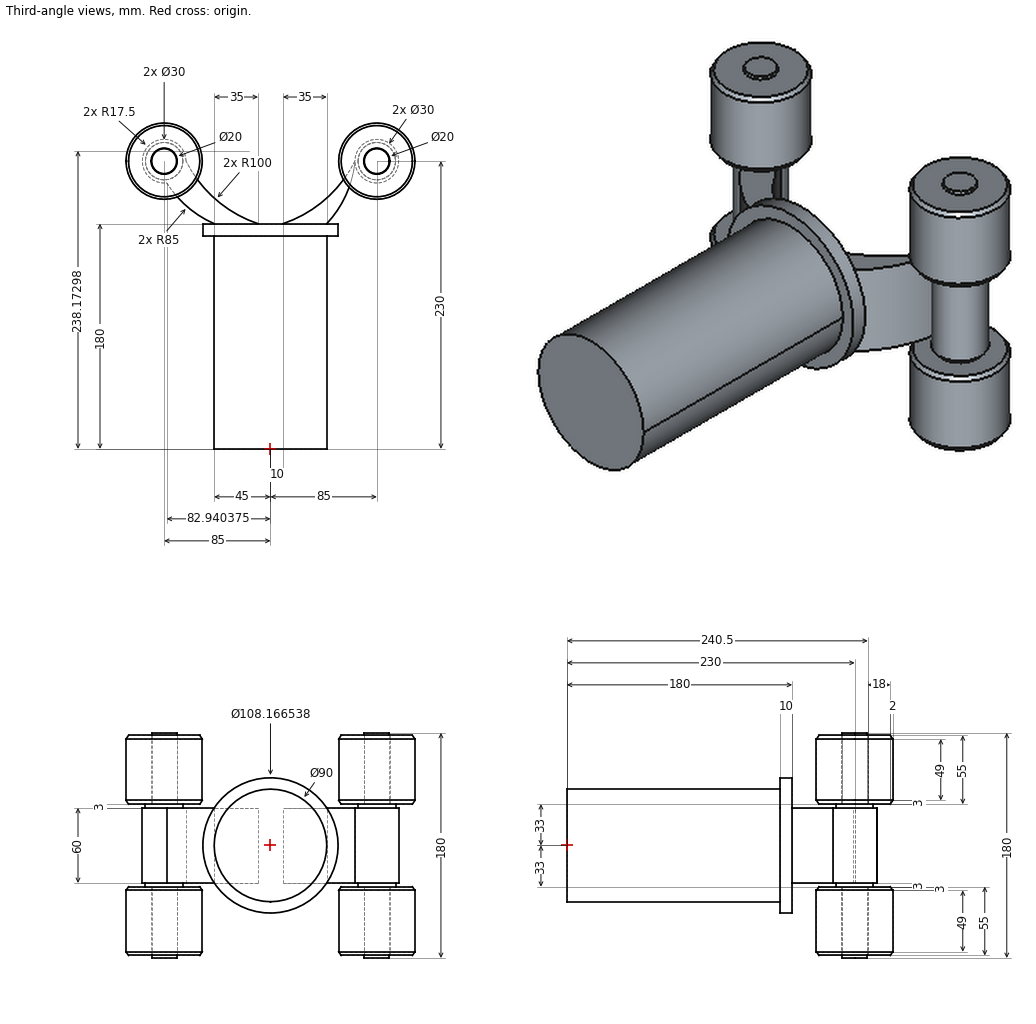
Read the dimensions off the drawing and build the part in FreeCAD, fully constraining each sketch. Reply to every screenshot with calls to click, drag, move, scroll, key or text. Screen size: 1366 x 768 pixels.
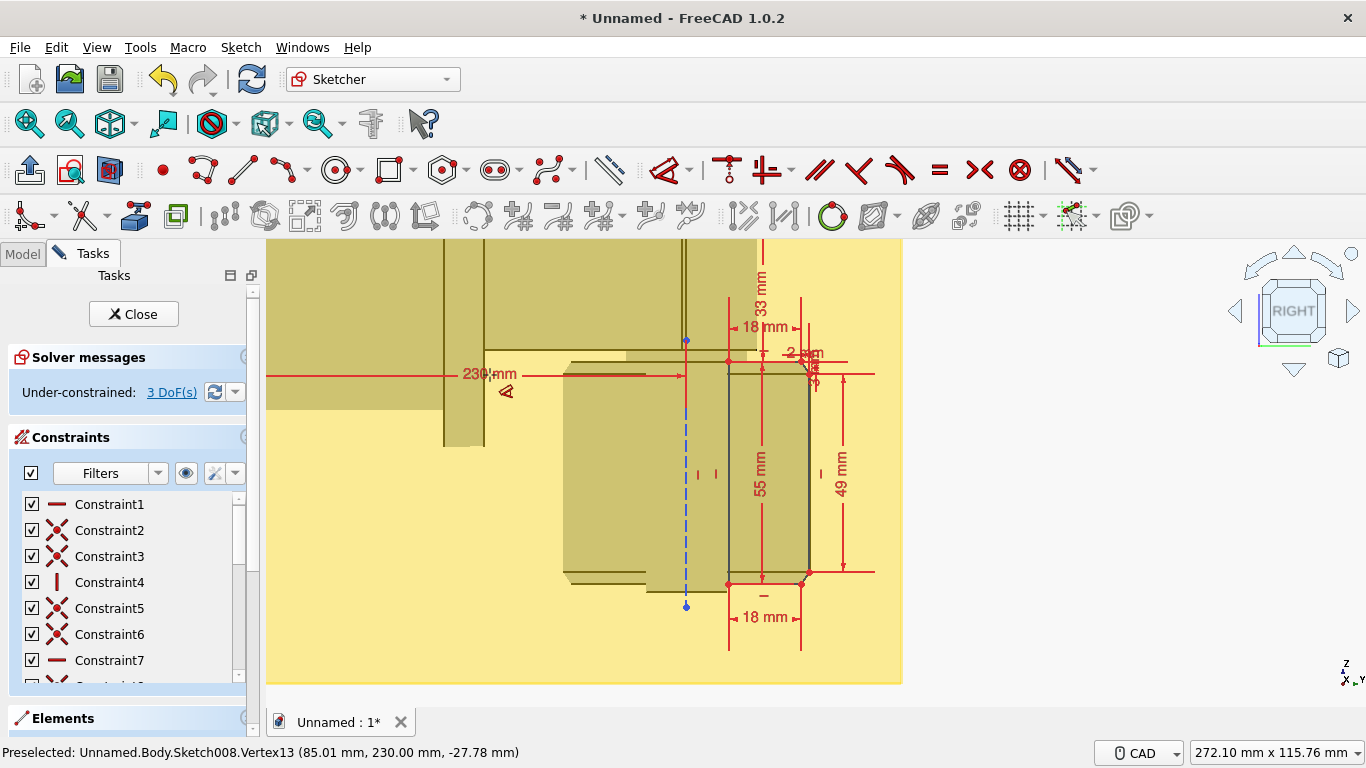
click(729, 362)
click(511, 396)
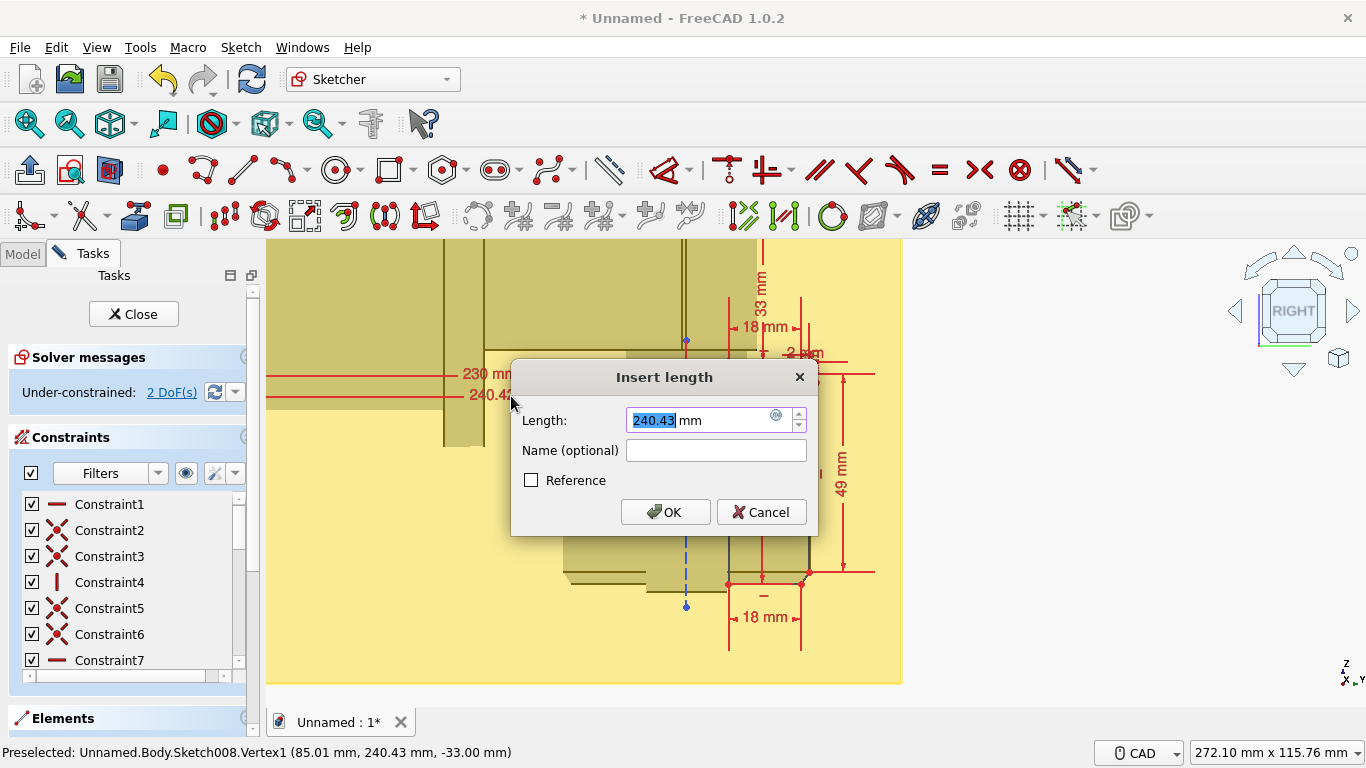
text(240.5)
key(Return)
key(Escape)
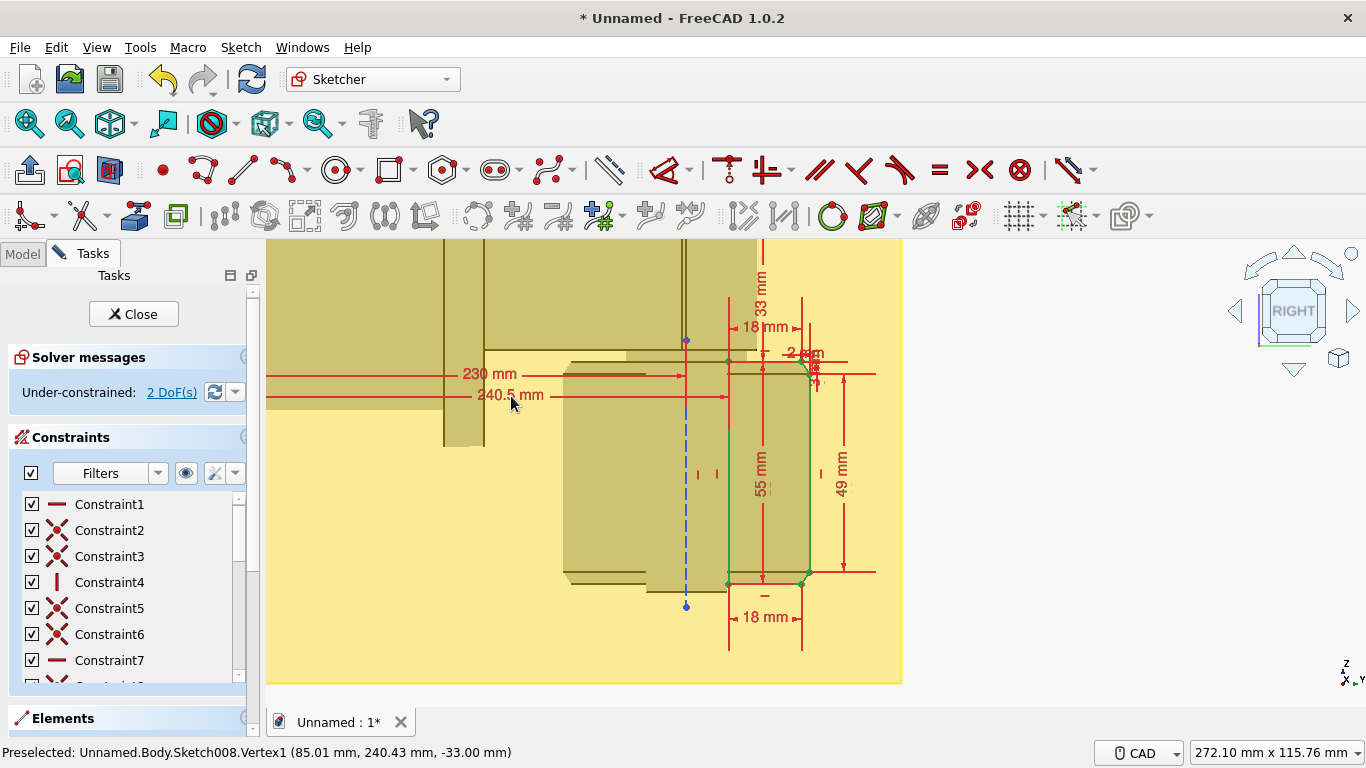
click(134, 314)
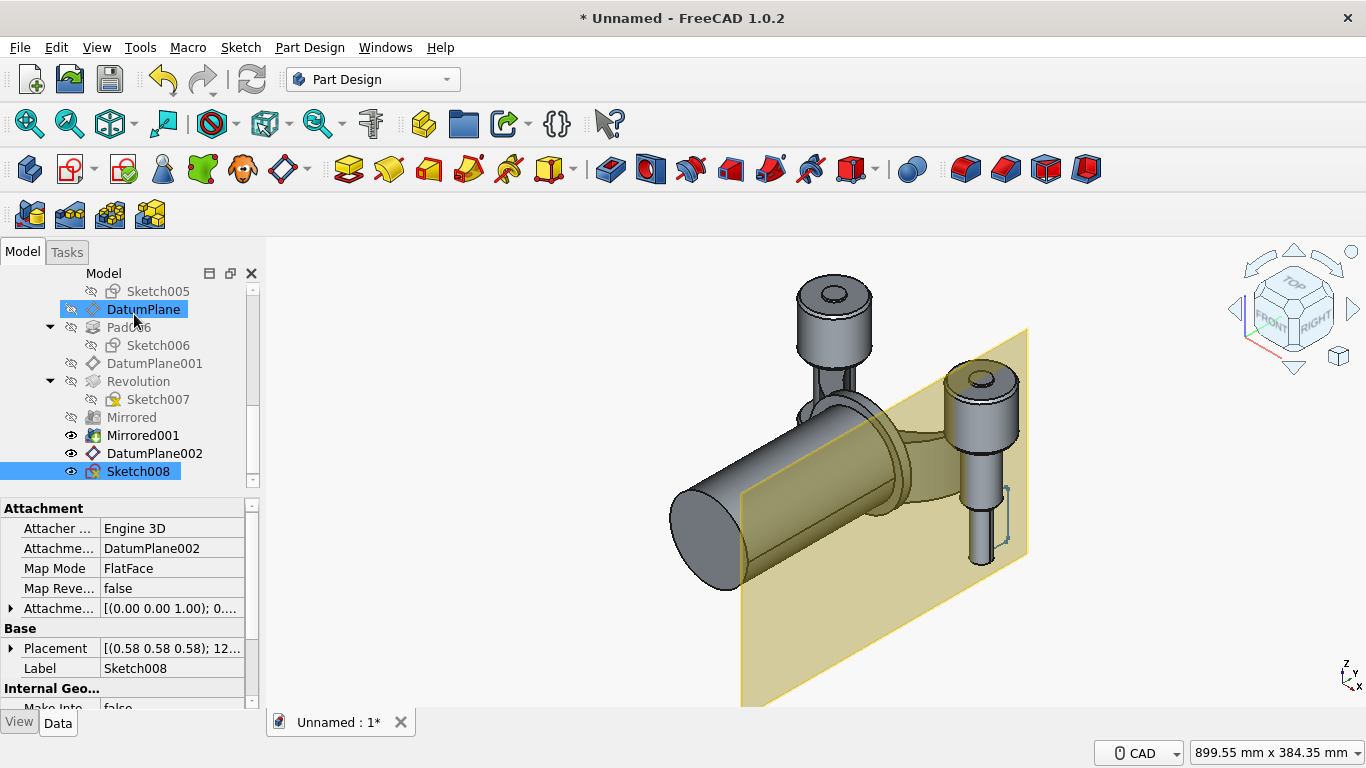
click(390, 170)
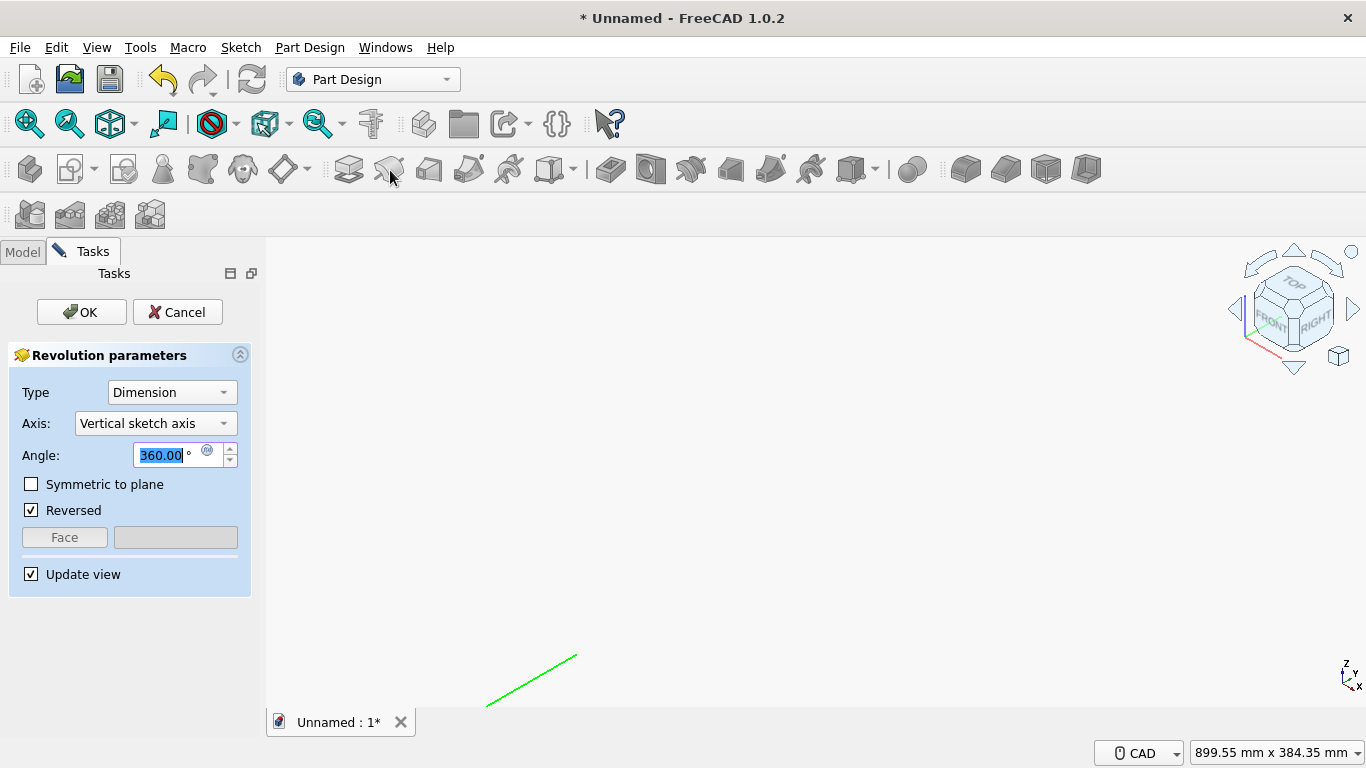
click(156, 424)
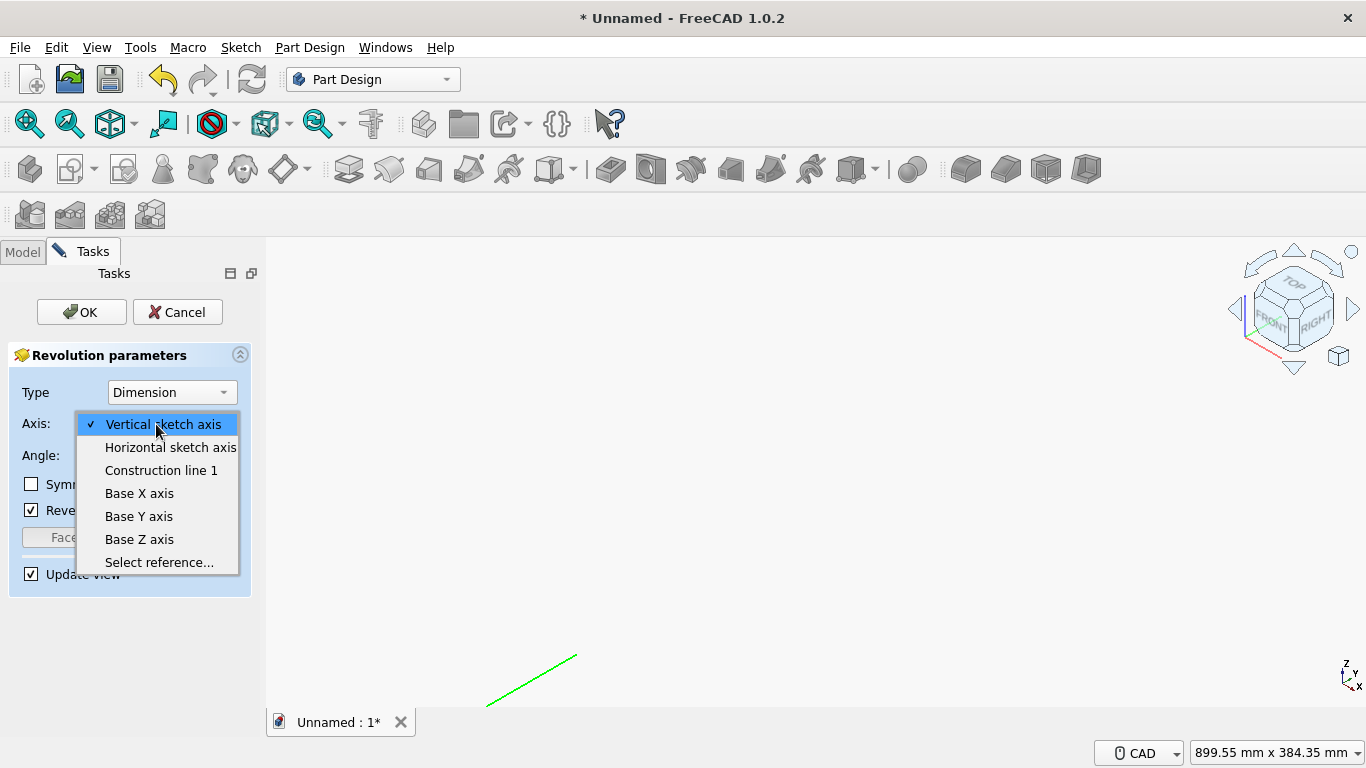
click(156, 470)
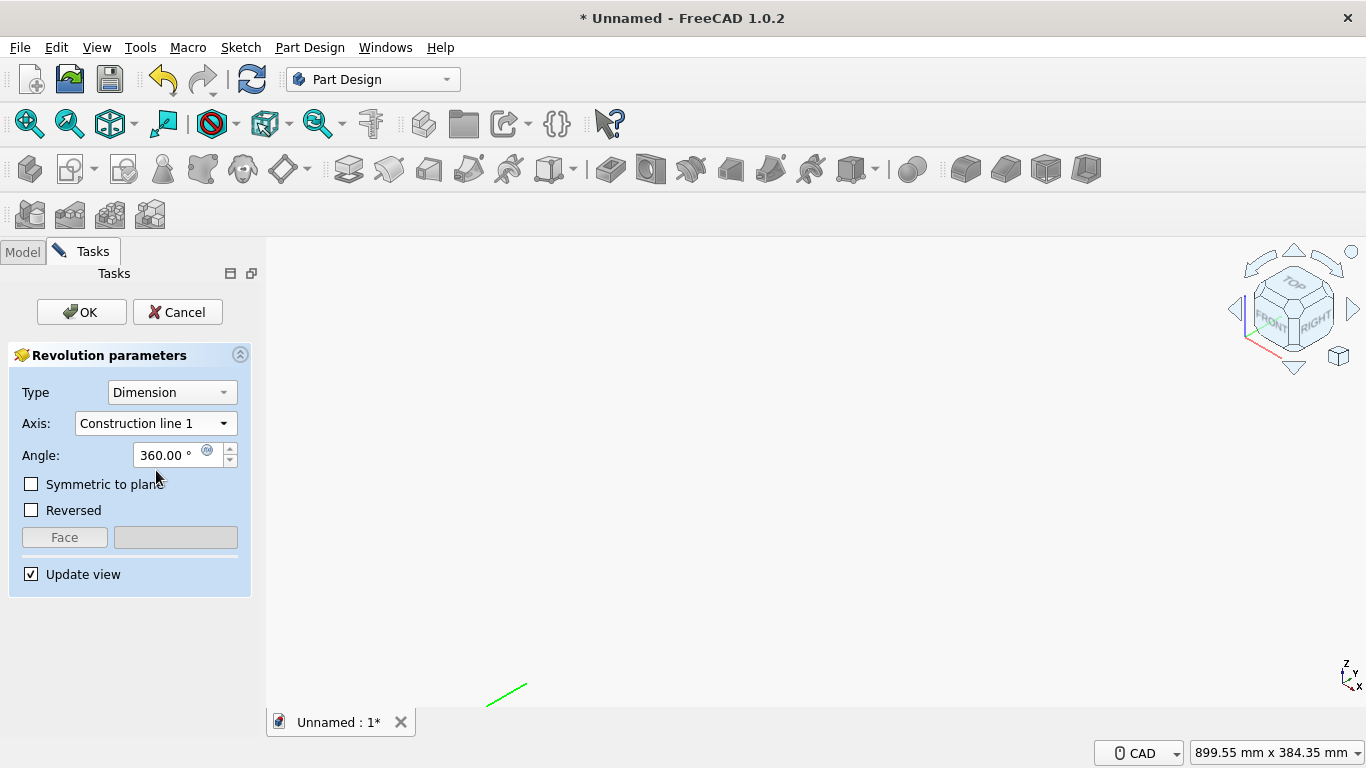
click(82, 312)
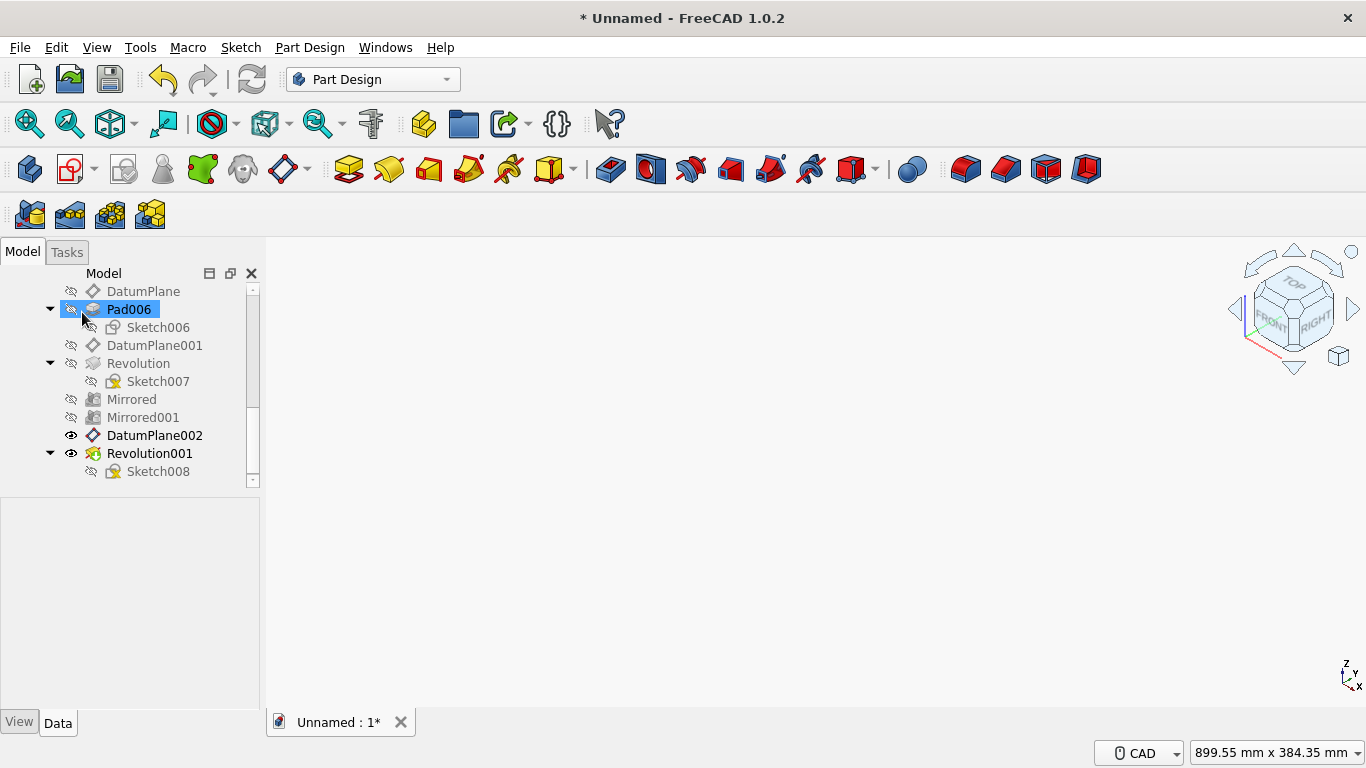
click(116, 435)
key(space)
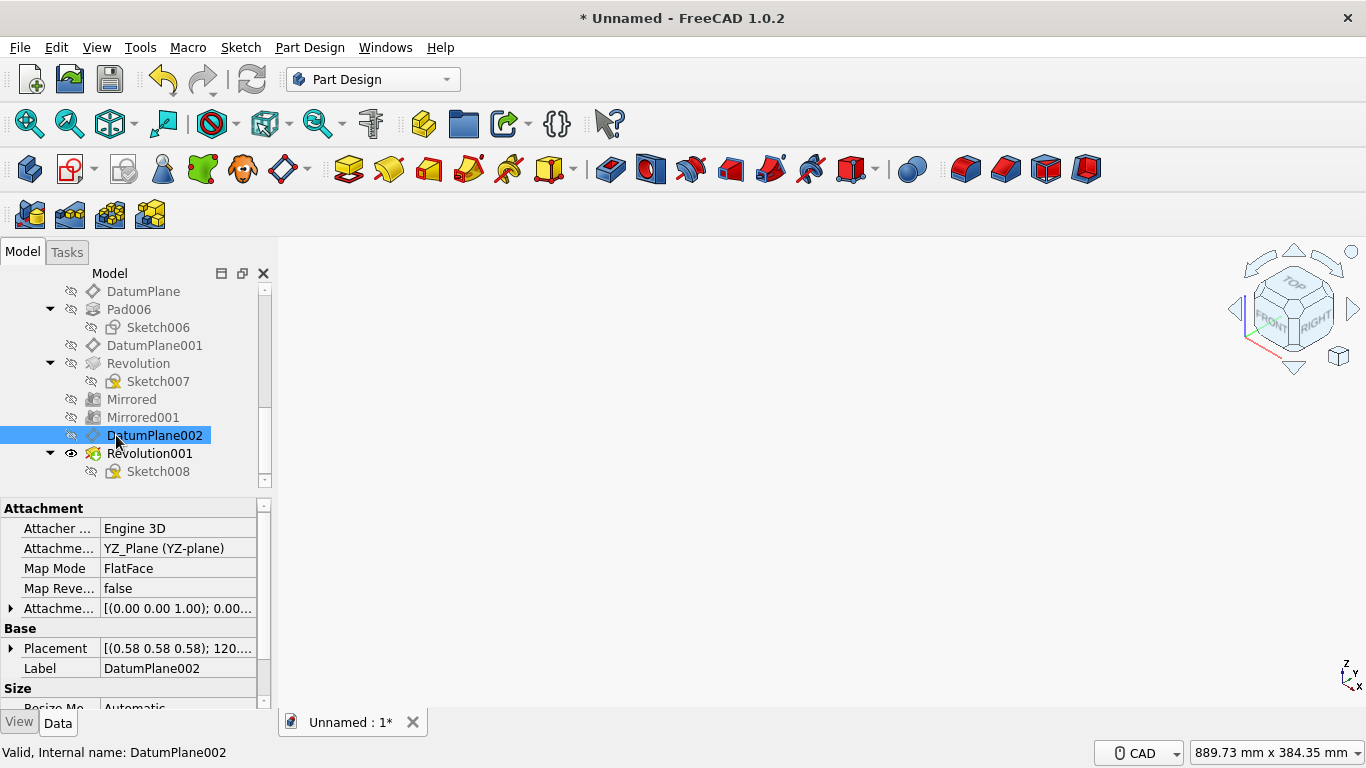
click(30, 124)